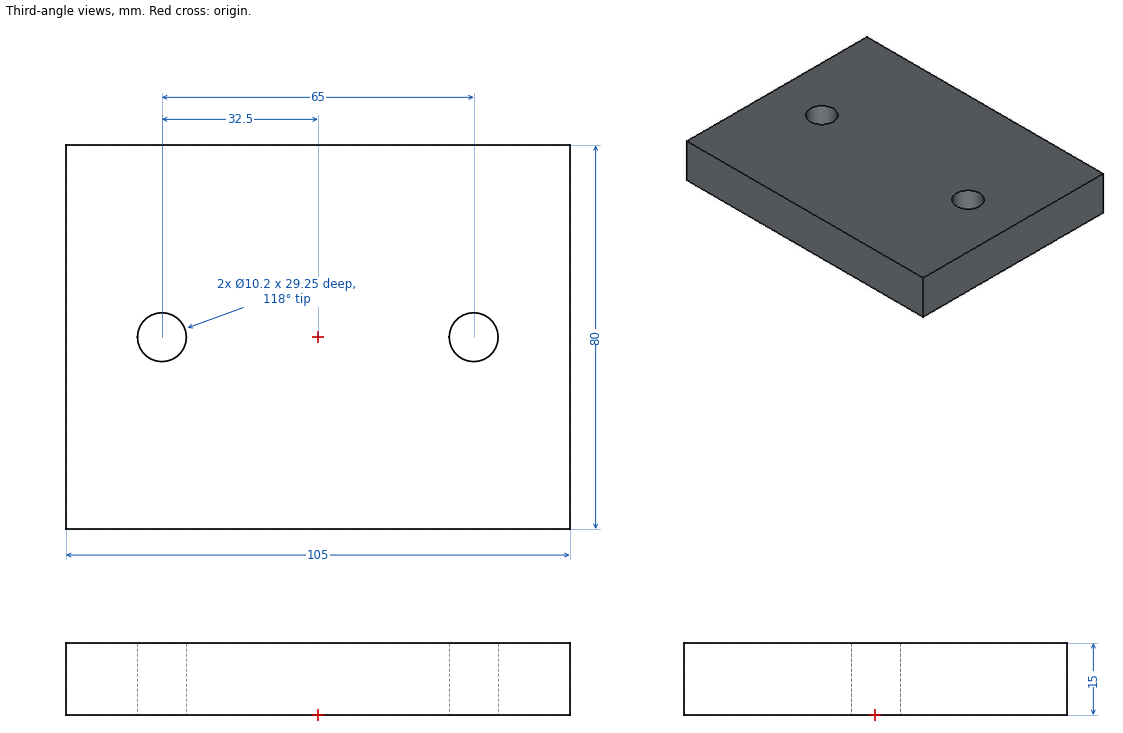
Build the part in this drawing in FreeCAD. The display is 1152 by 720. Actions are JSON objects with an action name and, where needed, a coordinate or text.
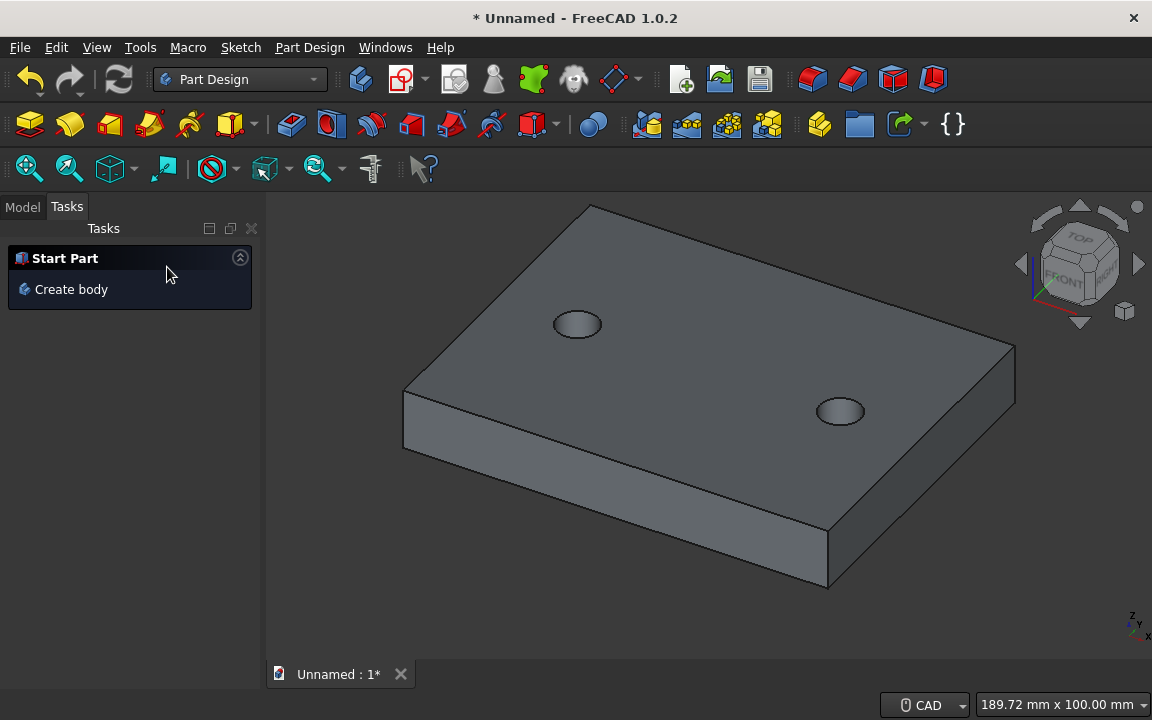
{"action": "key", "text": "0"}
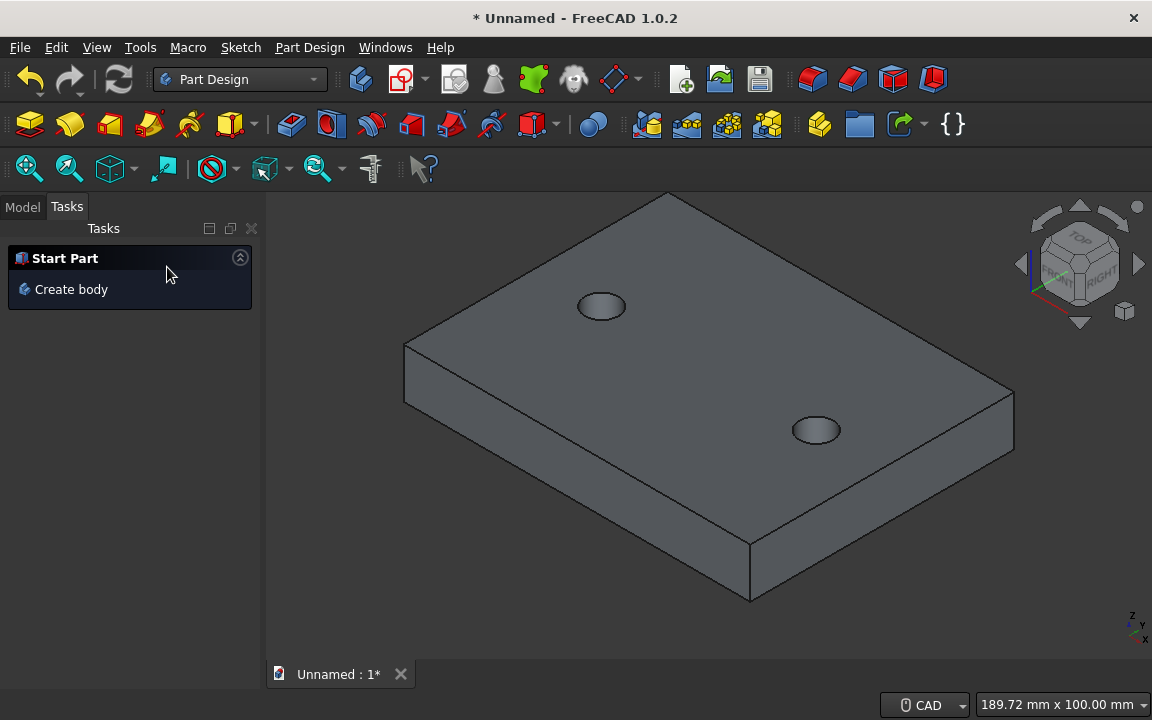
{"action": "left_click", "coordinate": [30, 170]}